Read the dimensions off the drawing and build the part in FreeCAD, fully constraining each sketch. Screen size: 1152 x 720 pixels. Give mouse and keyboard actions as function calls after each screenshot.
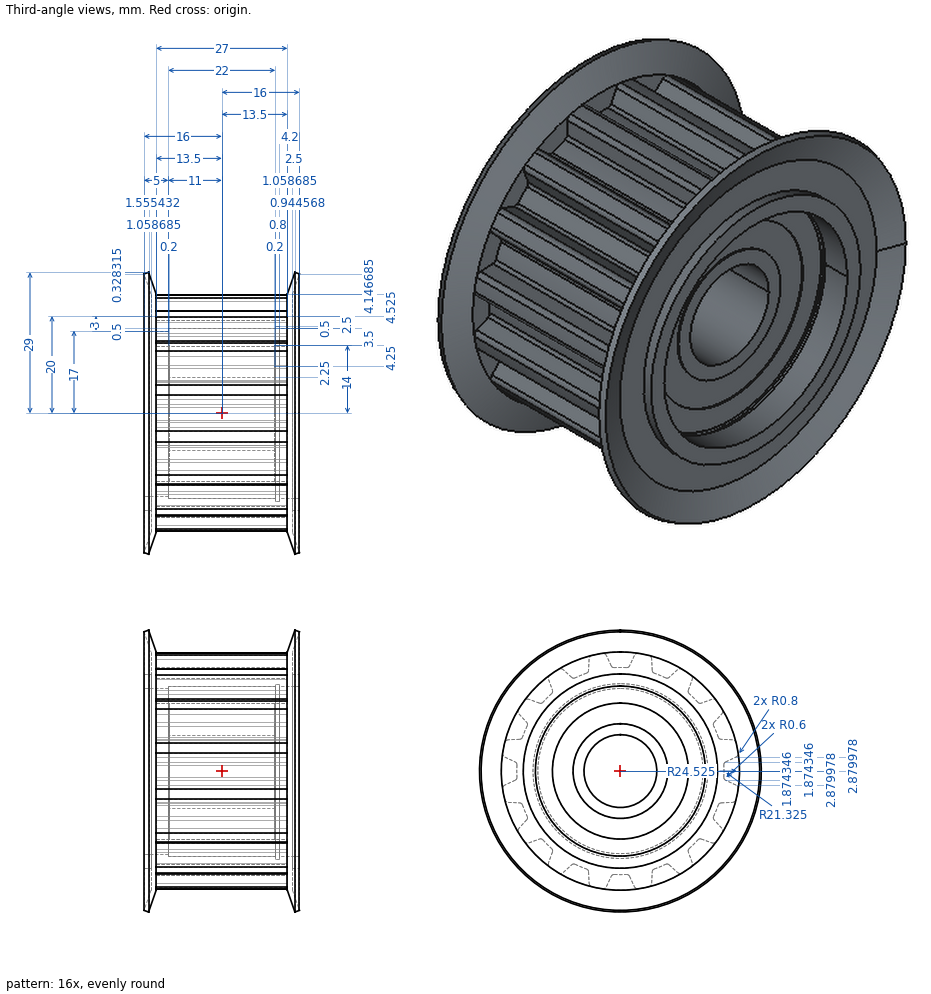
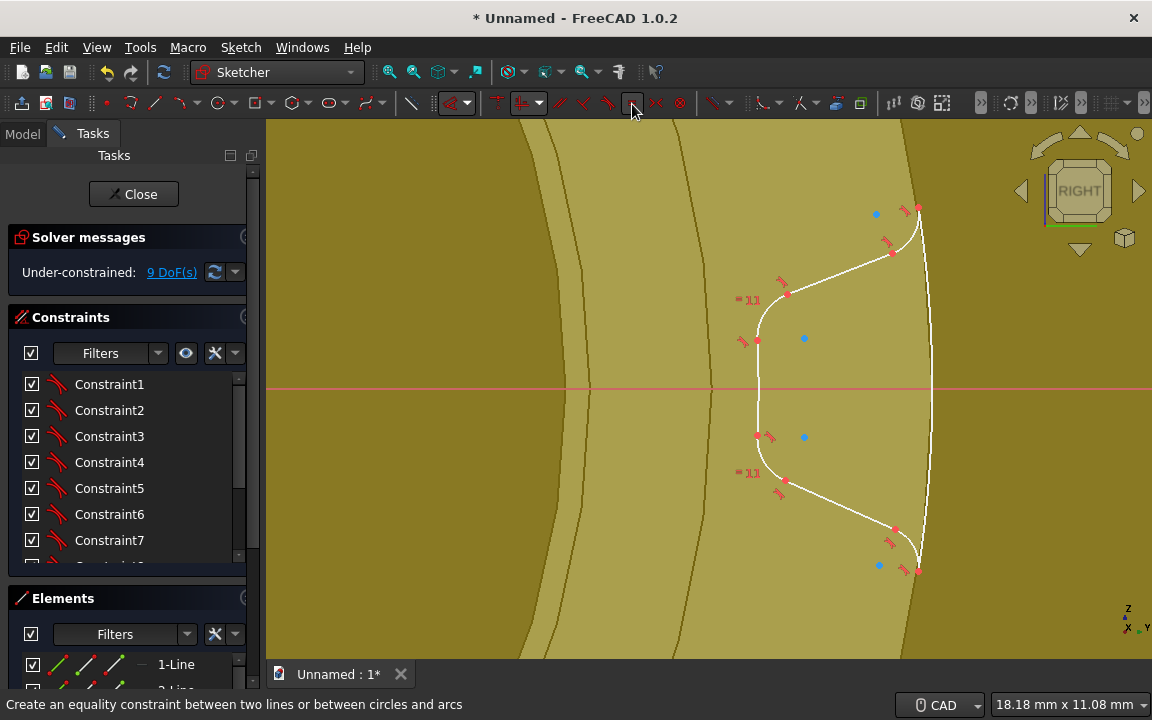
click(906, 244)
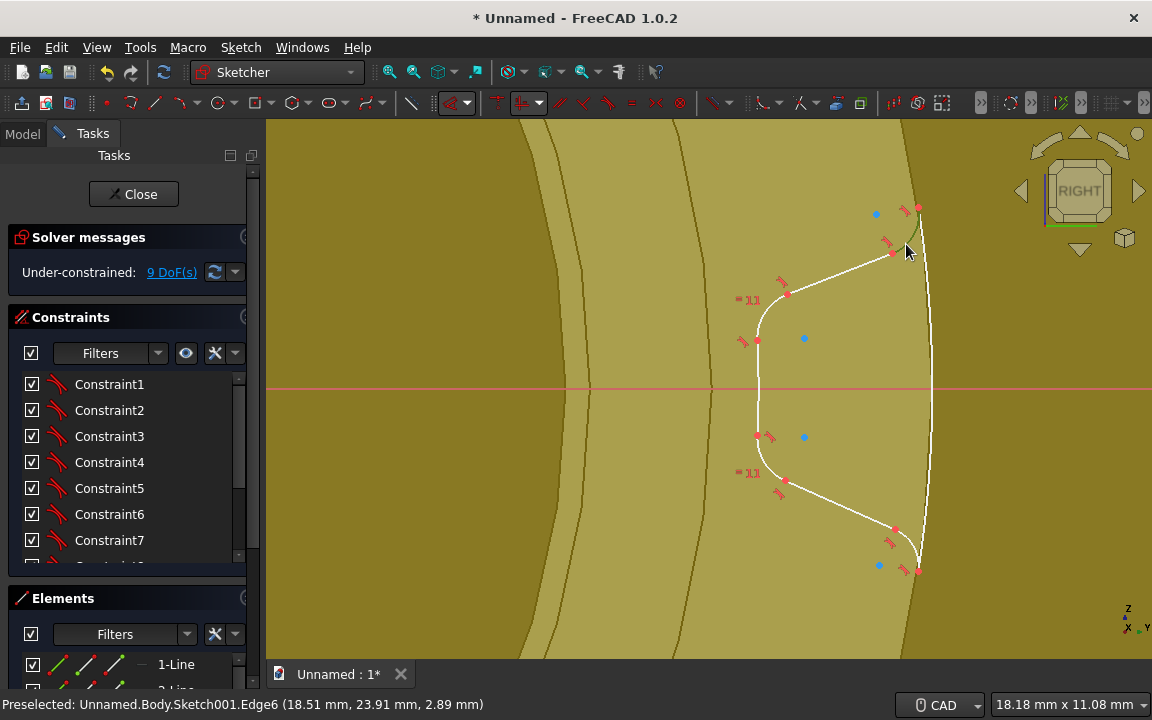
click(908, 539)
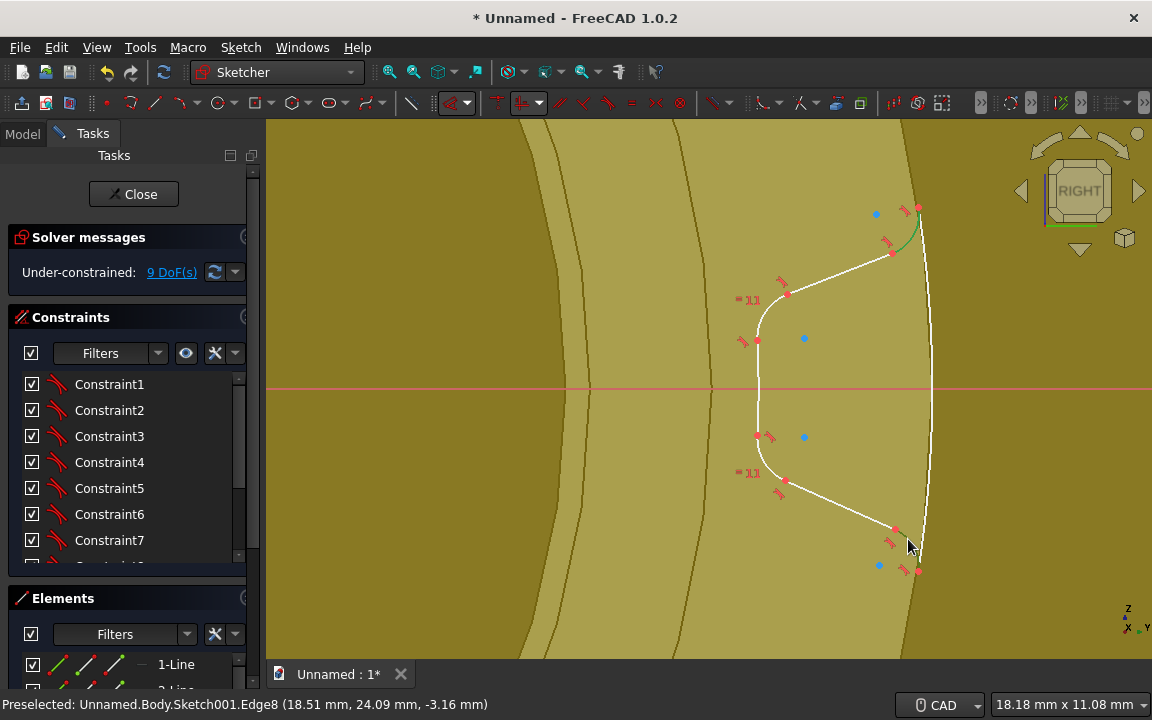
click(632, 104)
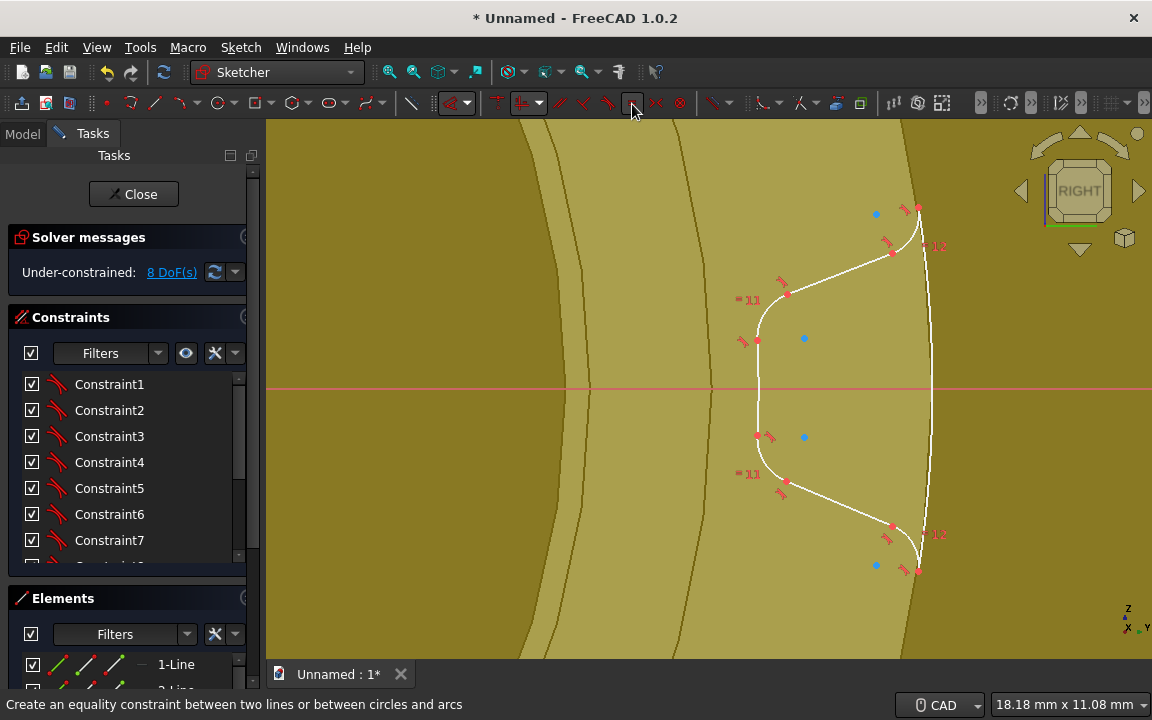
scroll(760, 453, up, 2)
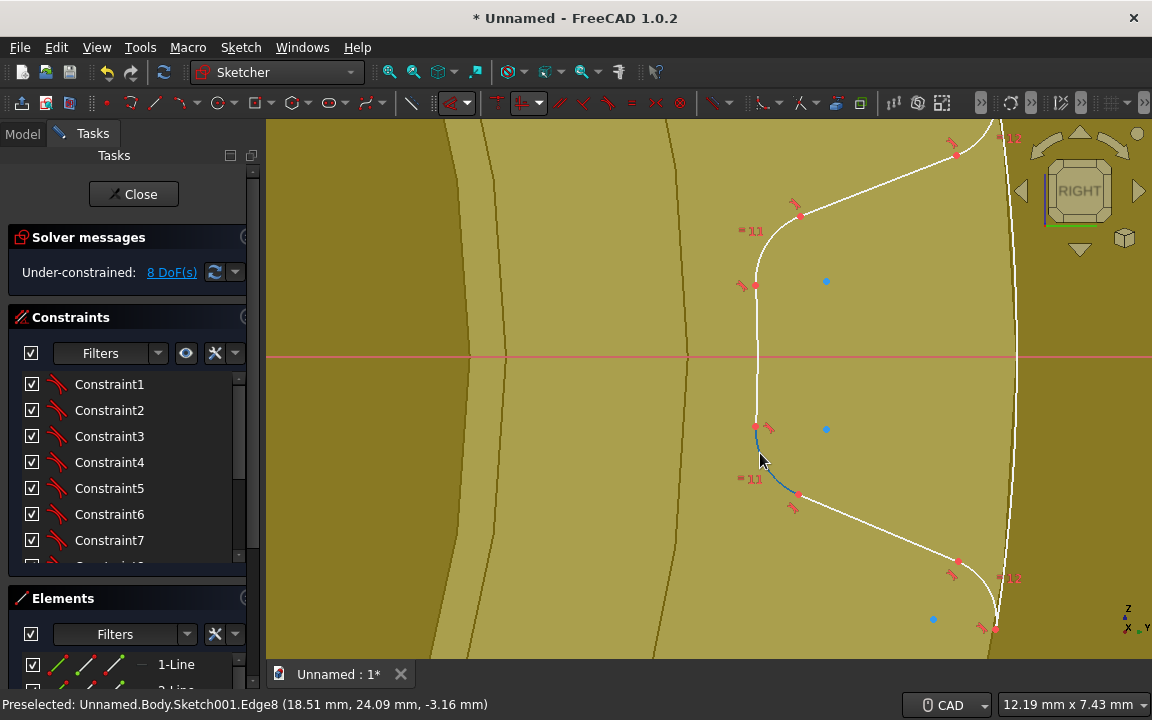
click(759, 452)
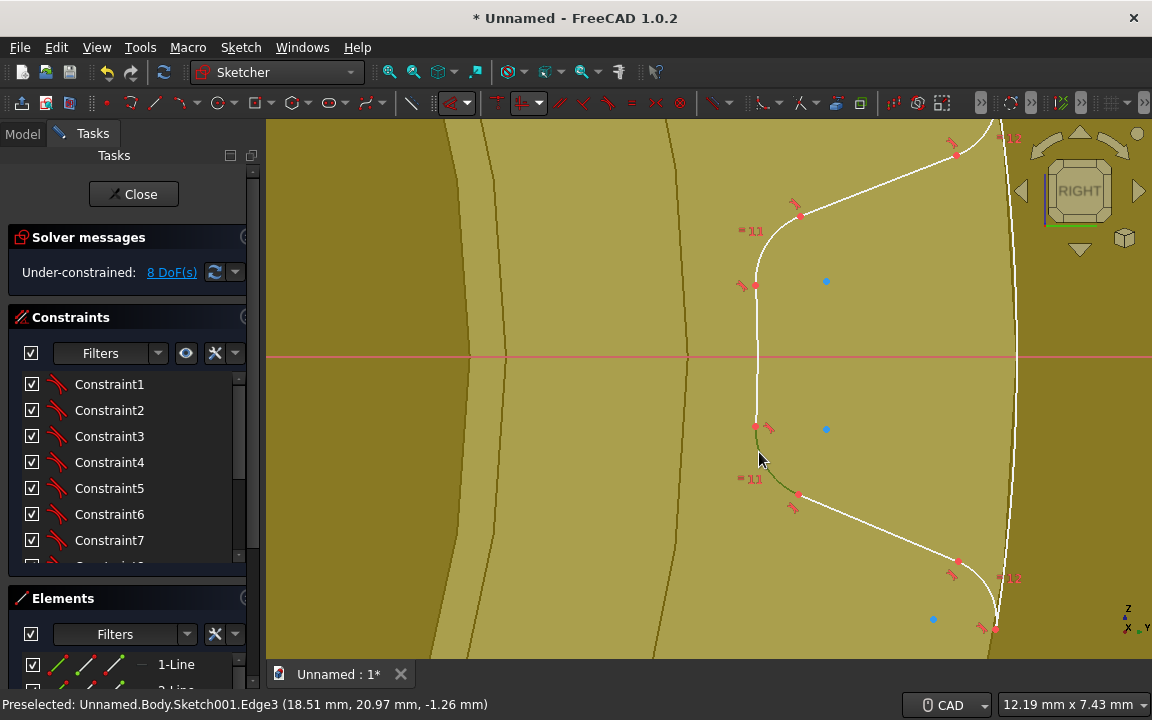
key(k)
key(r)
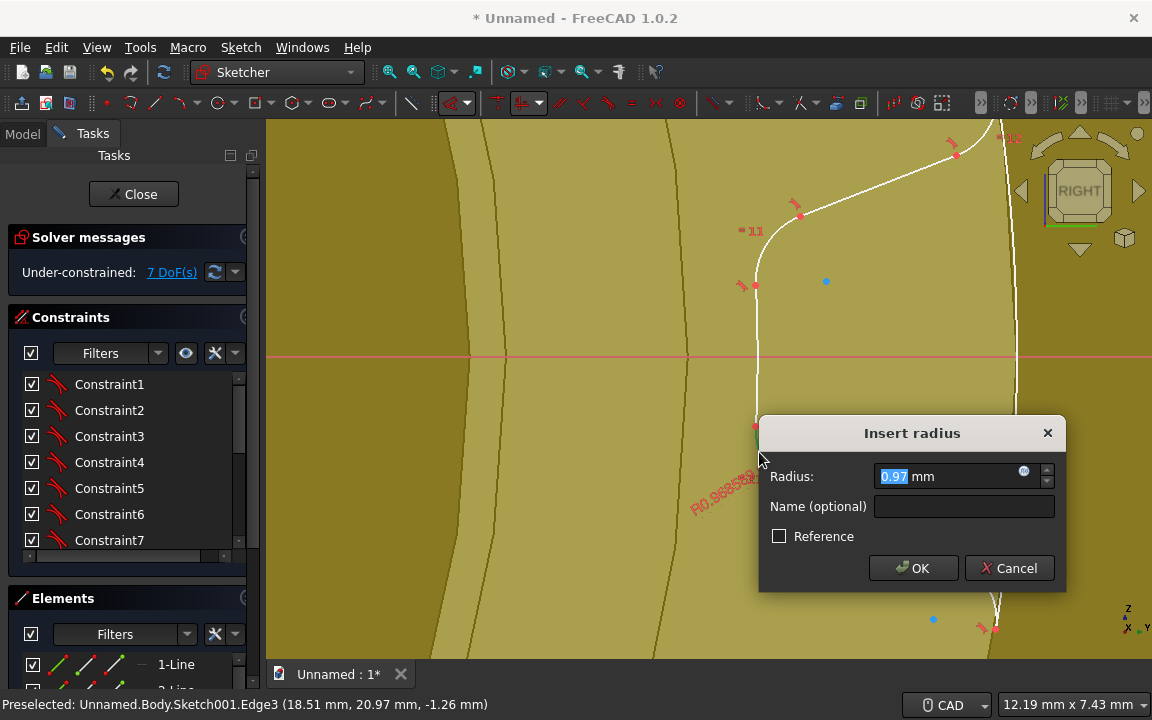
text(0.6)
key(Return)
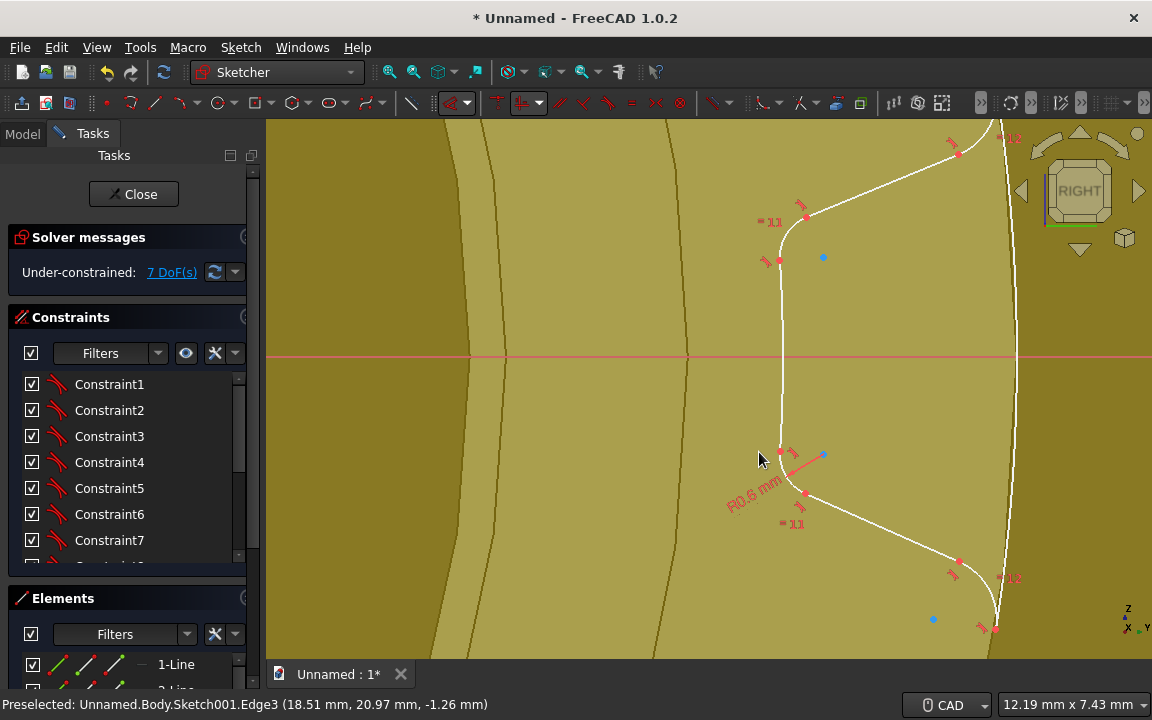
click(782, 394)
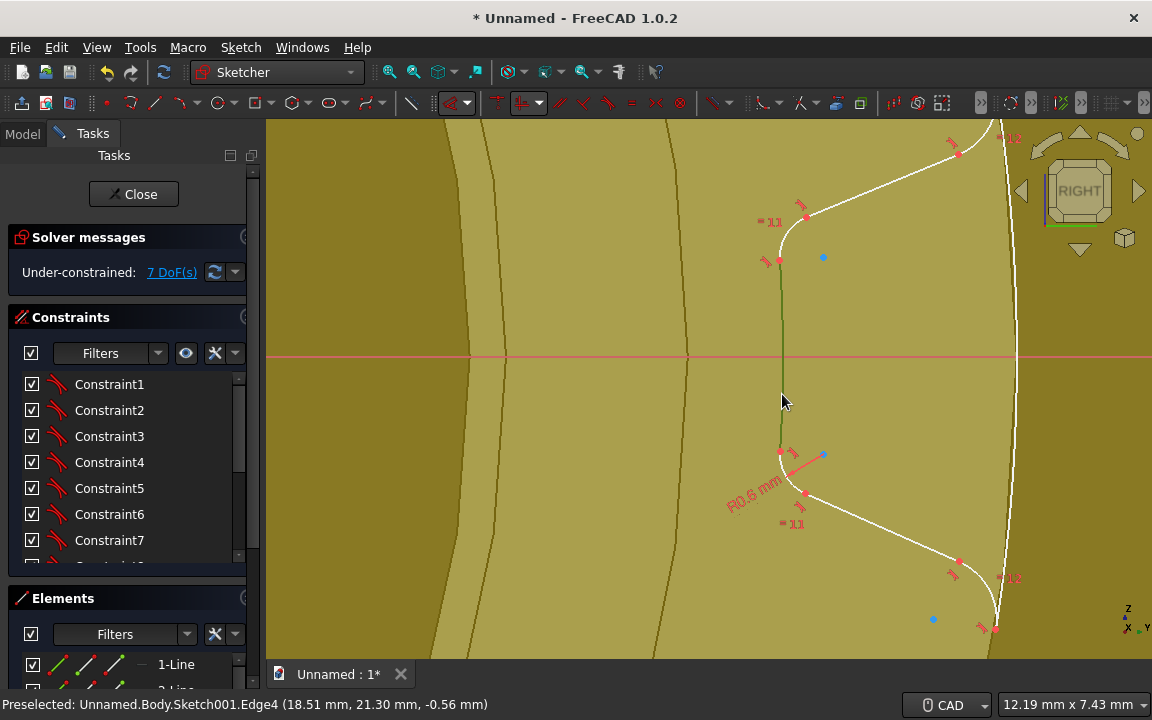
click(470, 104)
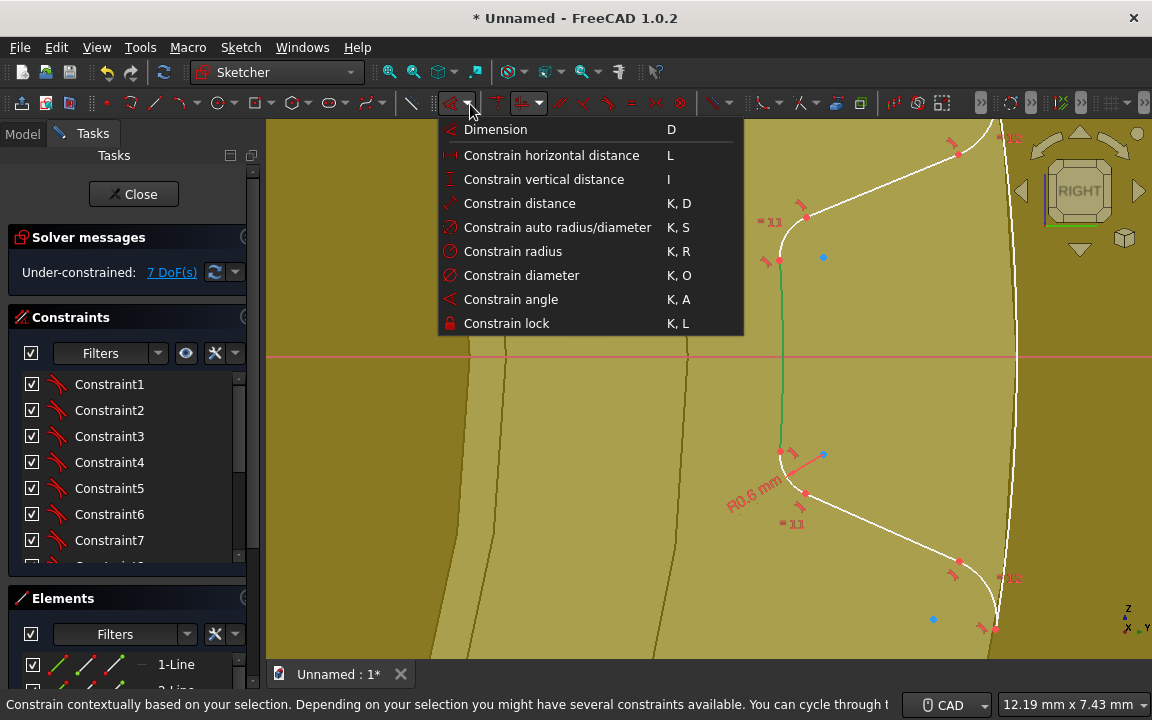
click(591, 251)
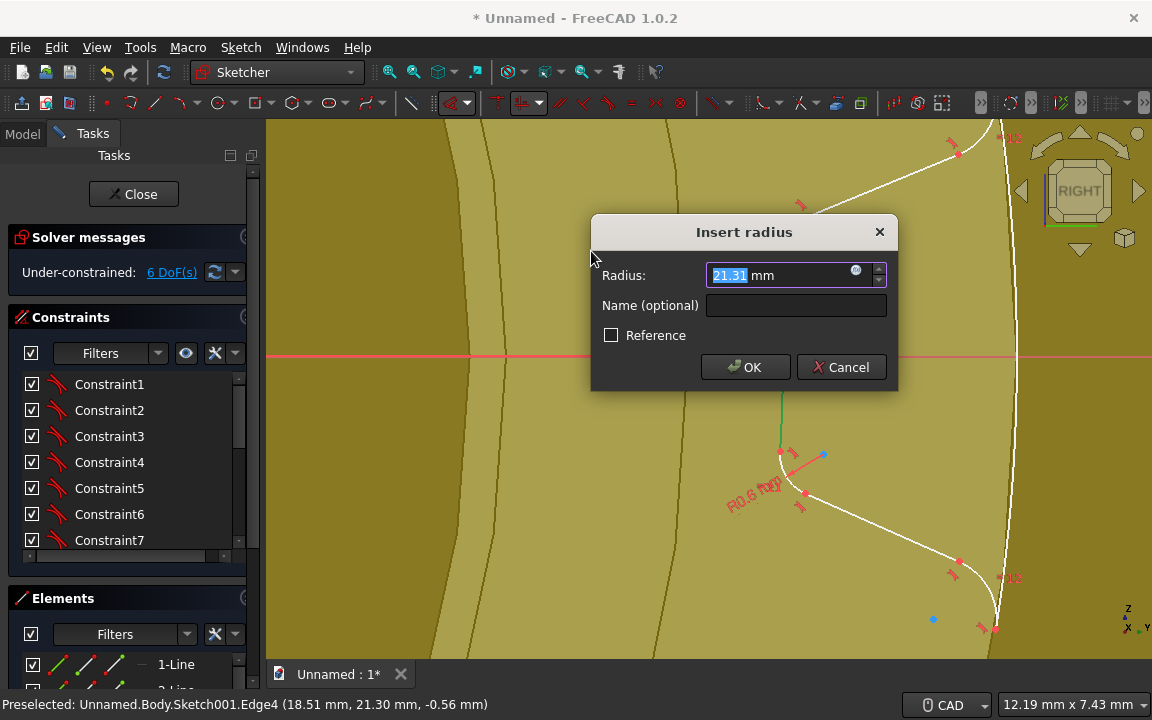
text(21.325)
key(Return)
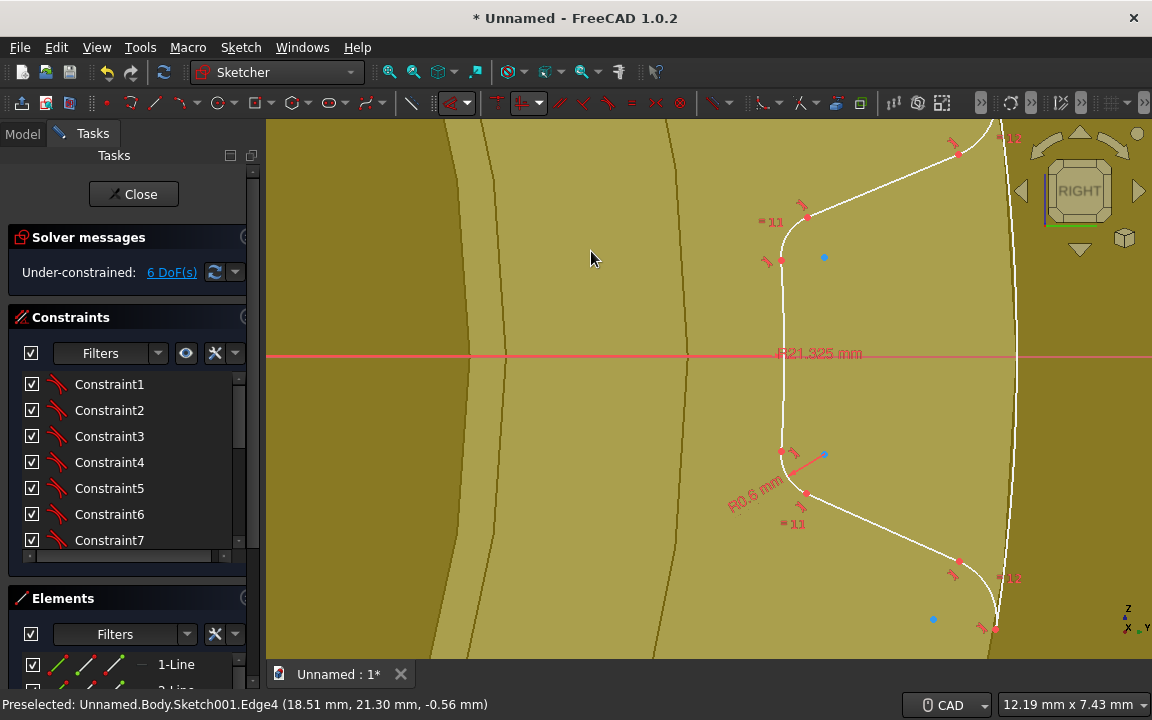
scroll(294, 454, down, 2)